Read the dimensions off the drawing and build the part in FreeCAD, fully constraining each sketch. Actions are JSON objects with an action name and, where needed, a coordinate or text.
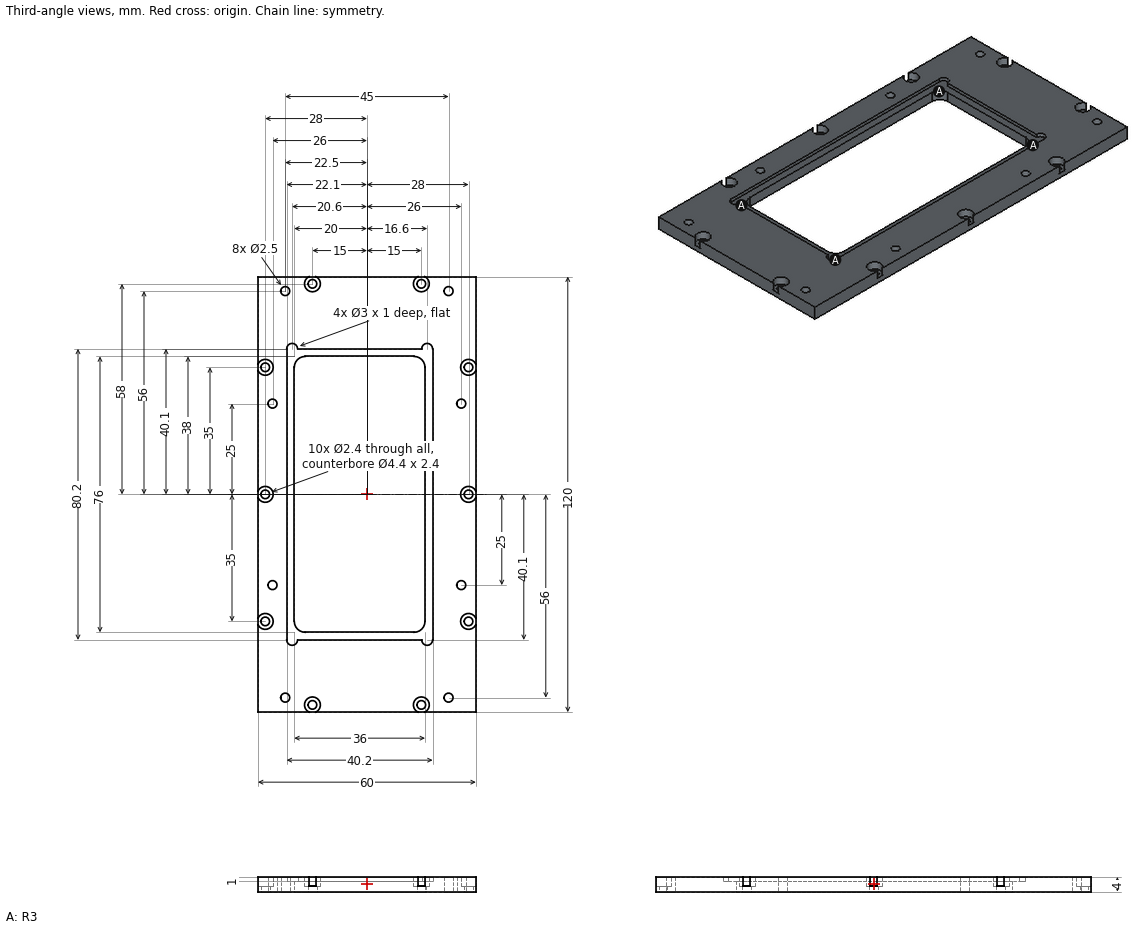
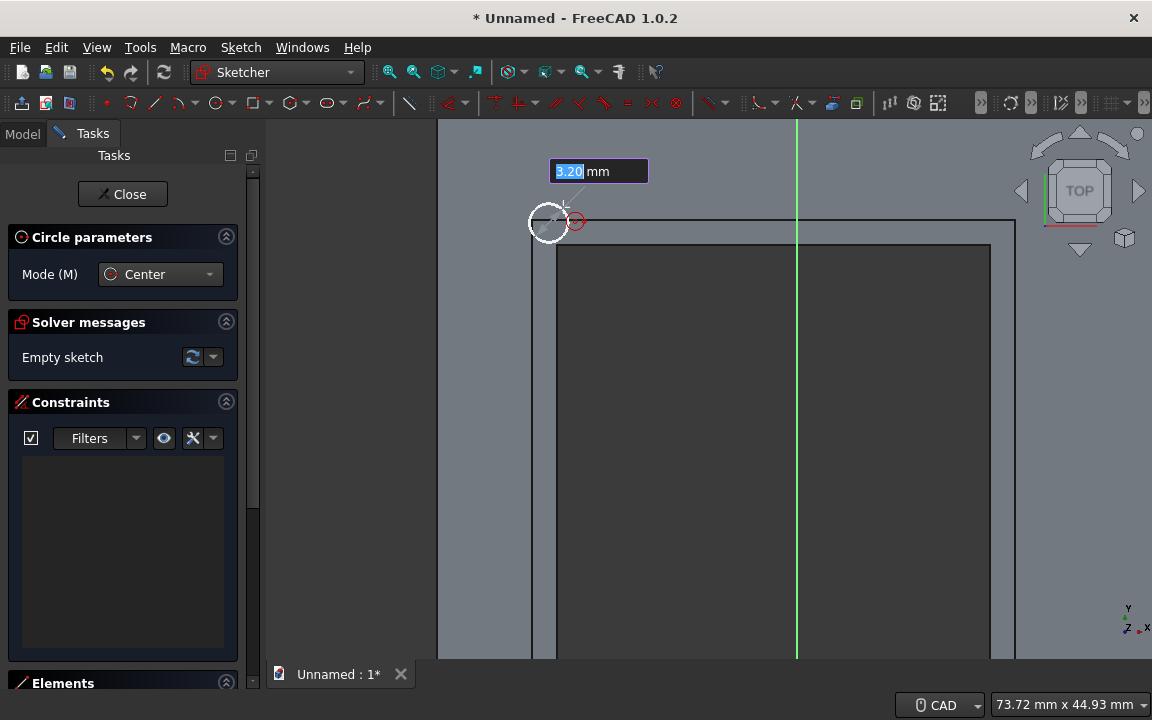
{"action": "left_click", "coordinate": [562, 207]}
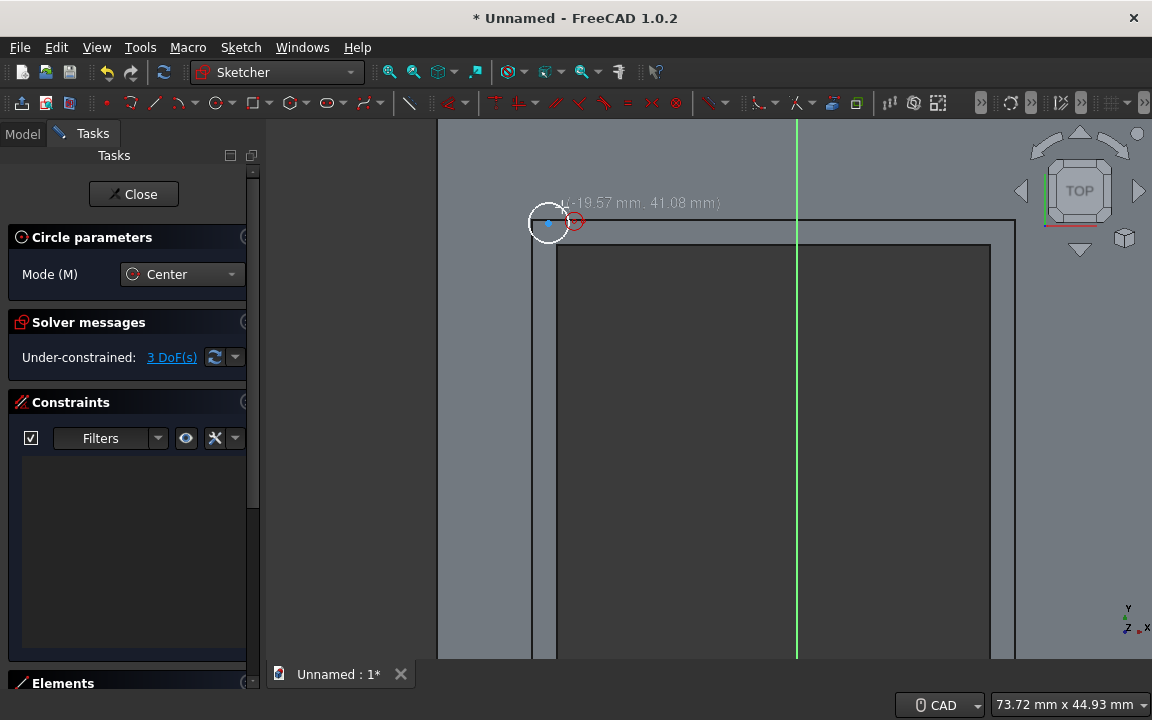
{"action": "scroll", "coordinate": [563, 207], "scroll_direction": "down", "scroll_amount": 5}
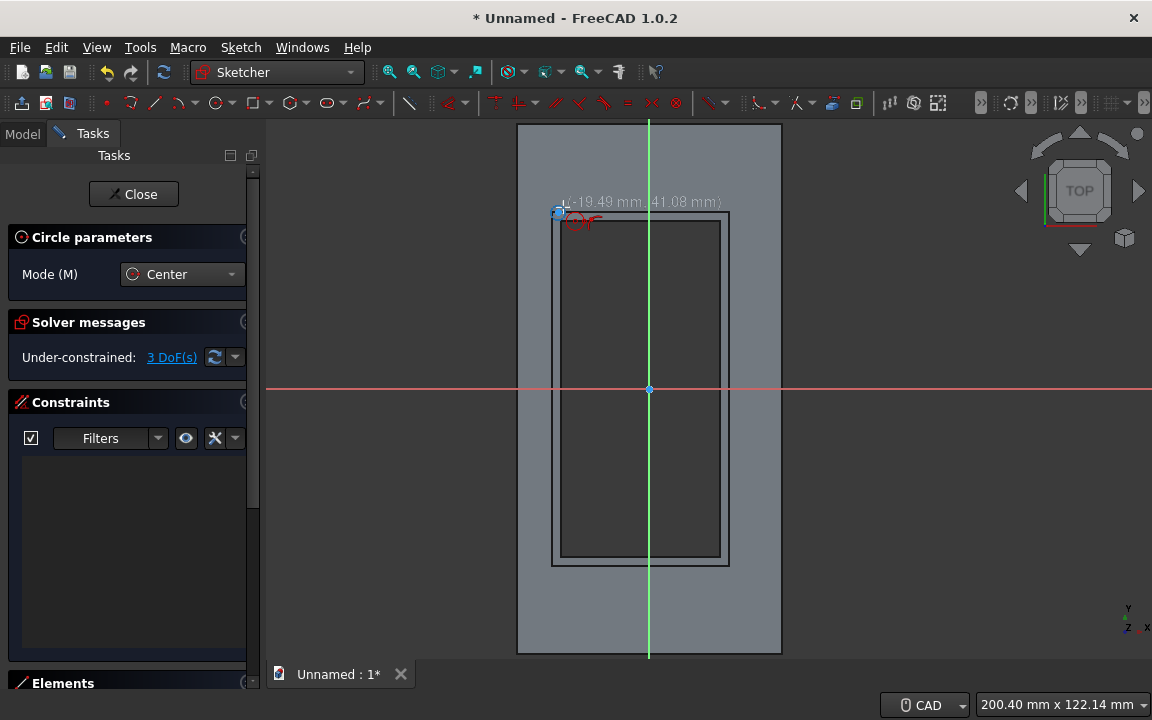
{"action": "scroll", "coordinate": [723, 212], "scroll_direction": "up", "scroll_amount": 7}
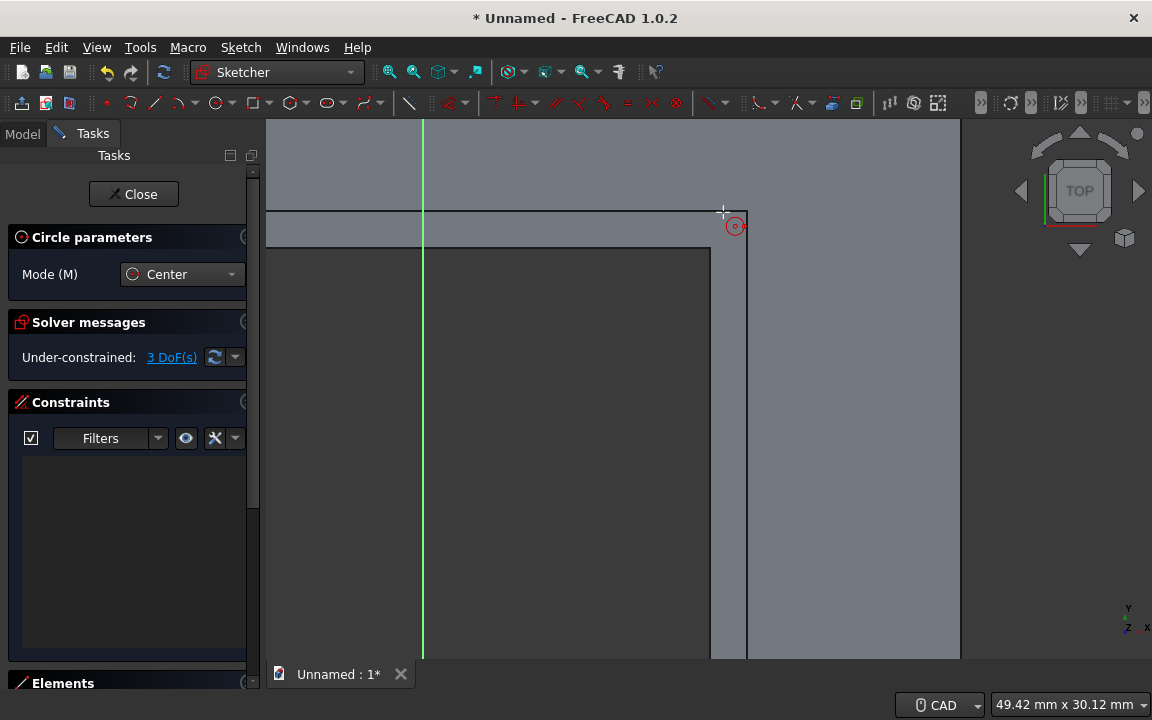
{"action": "scroll", "coordinate": [723, 212], "scroll_direction": "down", "scroll_amount": 7}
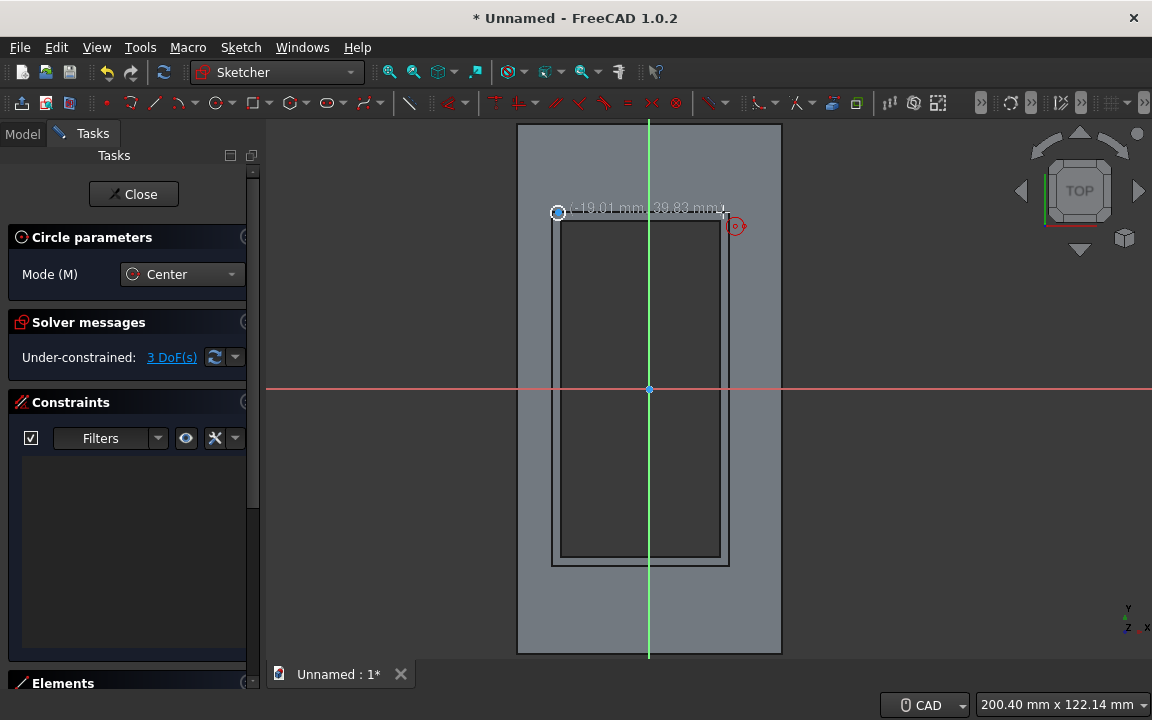
{"action": "left_click", "coordinate": [723, 212]}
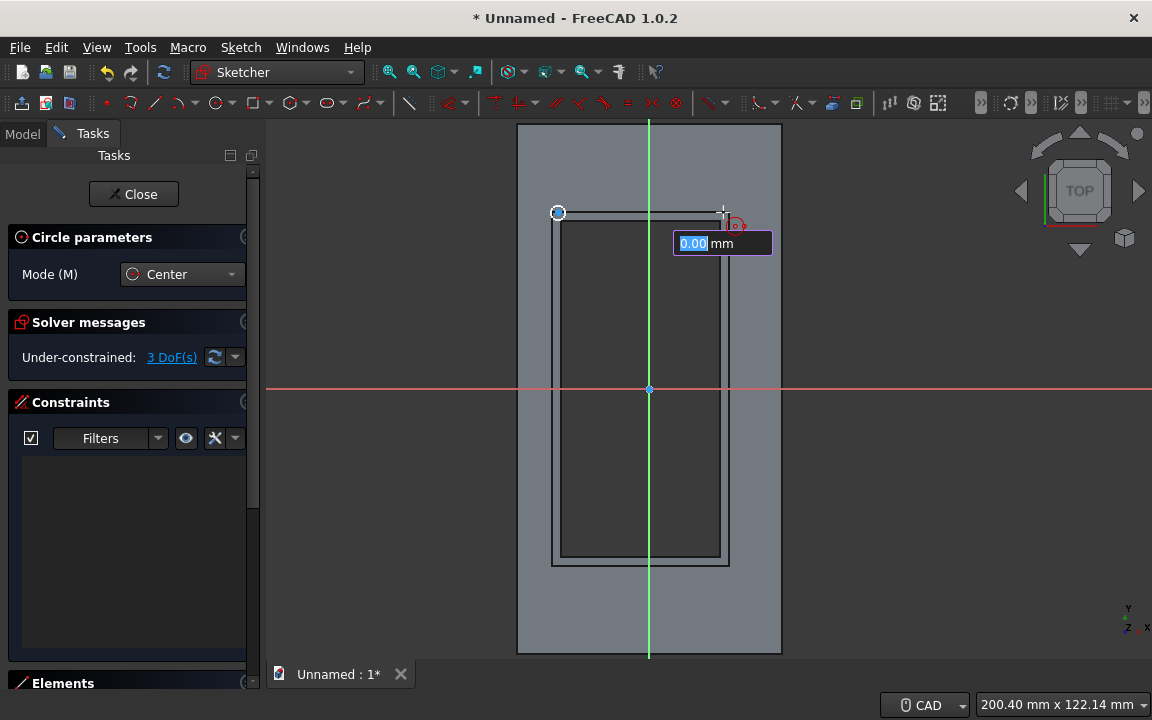
{"action": "scroll", "coordinate": [727, 207], "scroll_direction": "up", "scroll_amount": 5}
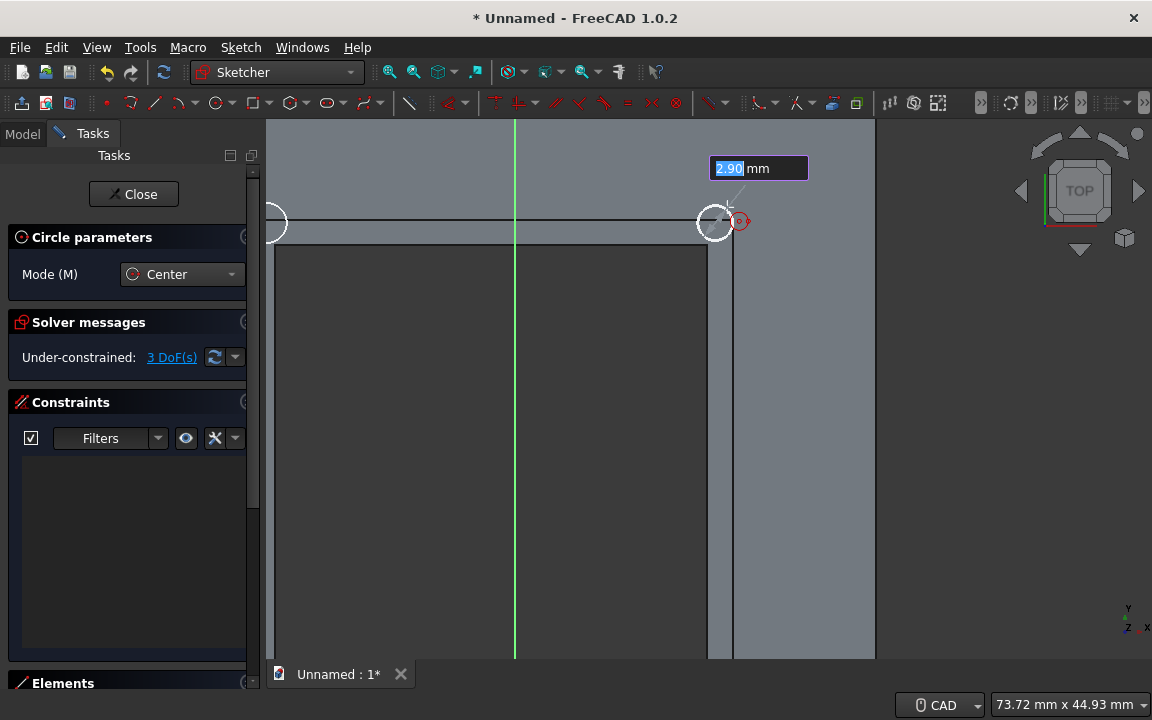
{"action": "left_click", "coordinate": [727, 207]}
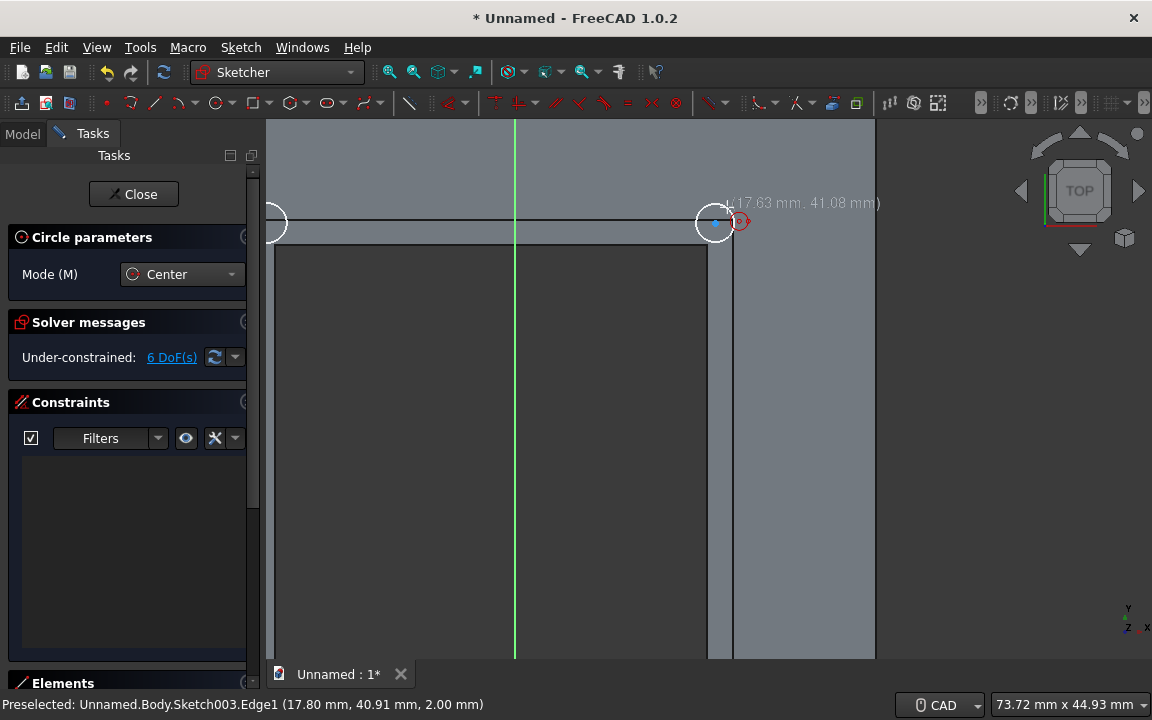
{"action": "scroll", "coordinate": [727, 207], "scroll_direction": "down", "scroll_amount": 5}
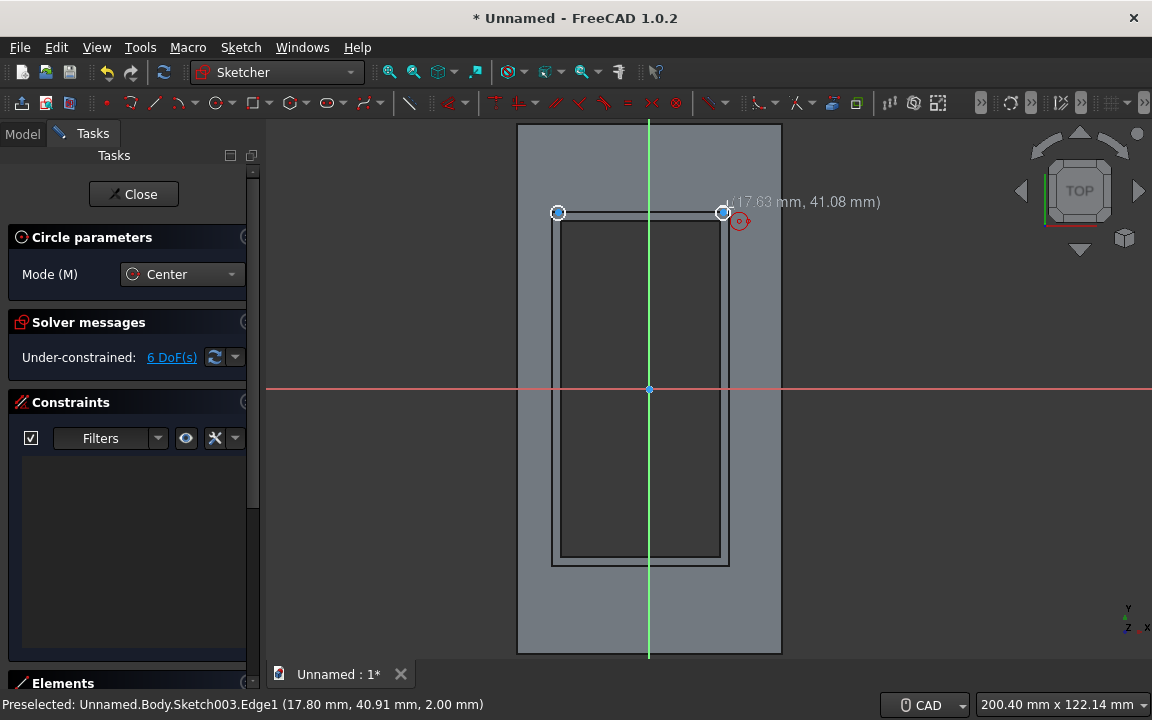
{"action": "scroll", "coordinate": [723, 566], "scroll_direction": "up", "scroll_amount": 7}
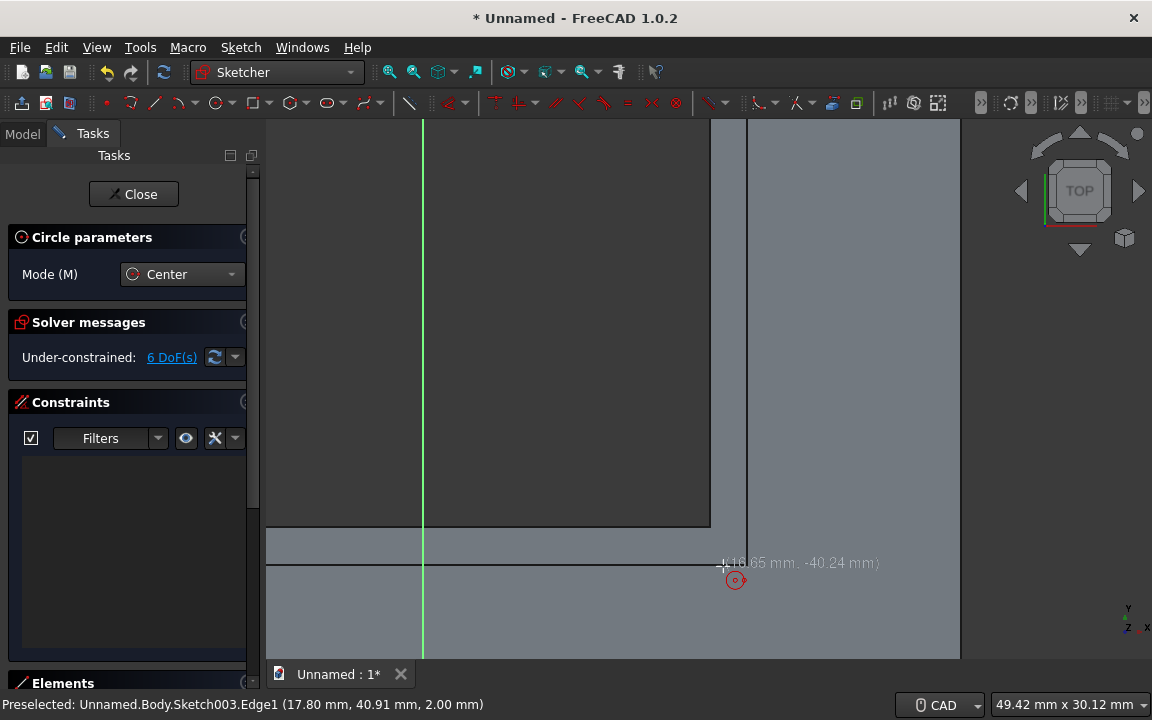
{"action": "scroll", "coordinate": [723, 567], "scroll_direction": "down", "scroll_amount": 7}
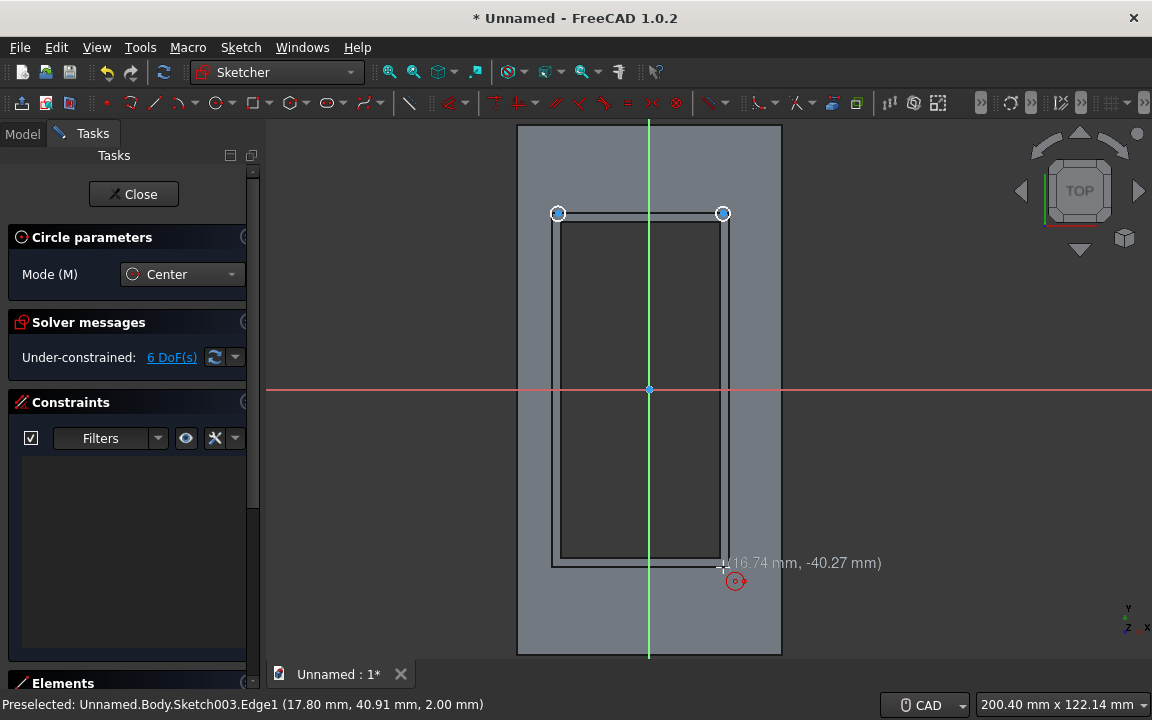
{"action": "left_click", "coordinate": [723, 567]}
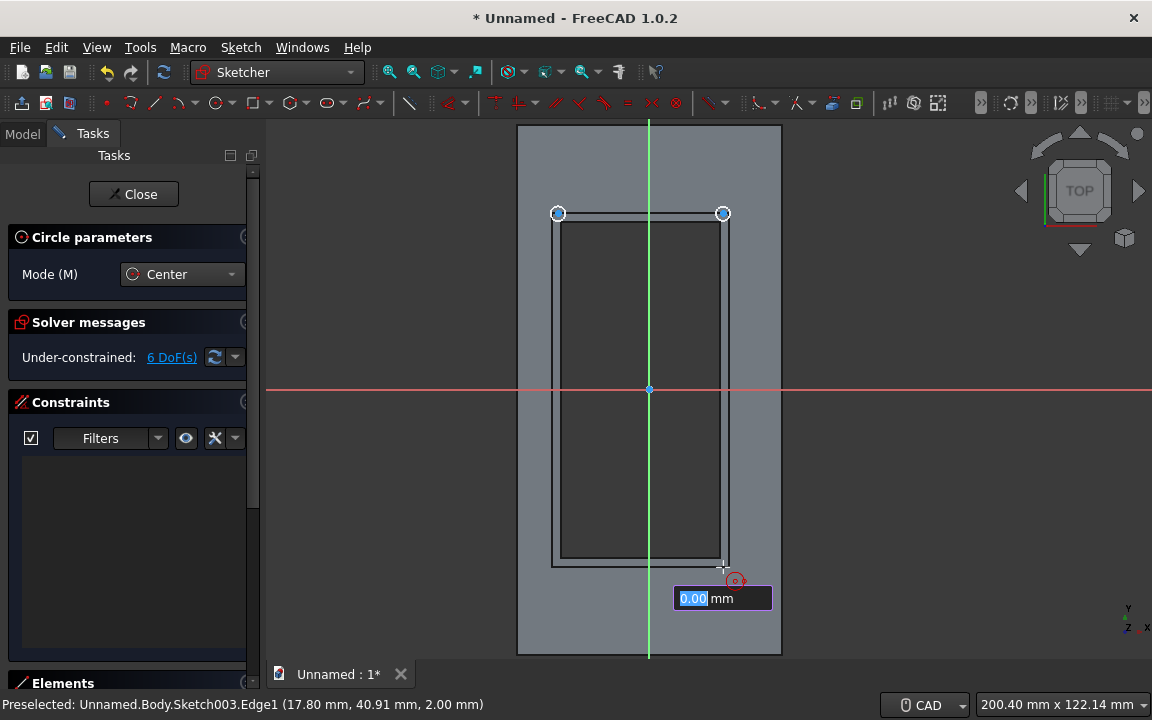
{"action": "scroll", "coordinate": [727, 562], "scroll_direction": "up", "scroll_amount": 5}